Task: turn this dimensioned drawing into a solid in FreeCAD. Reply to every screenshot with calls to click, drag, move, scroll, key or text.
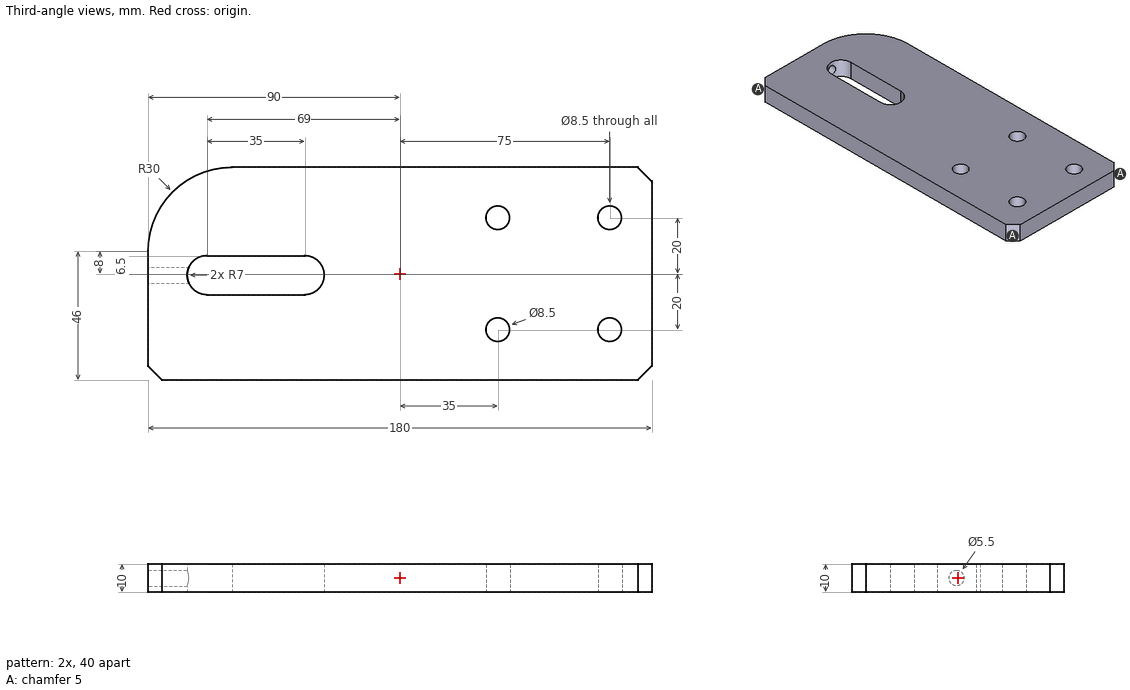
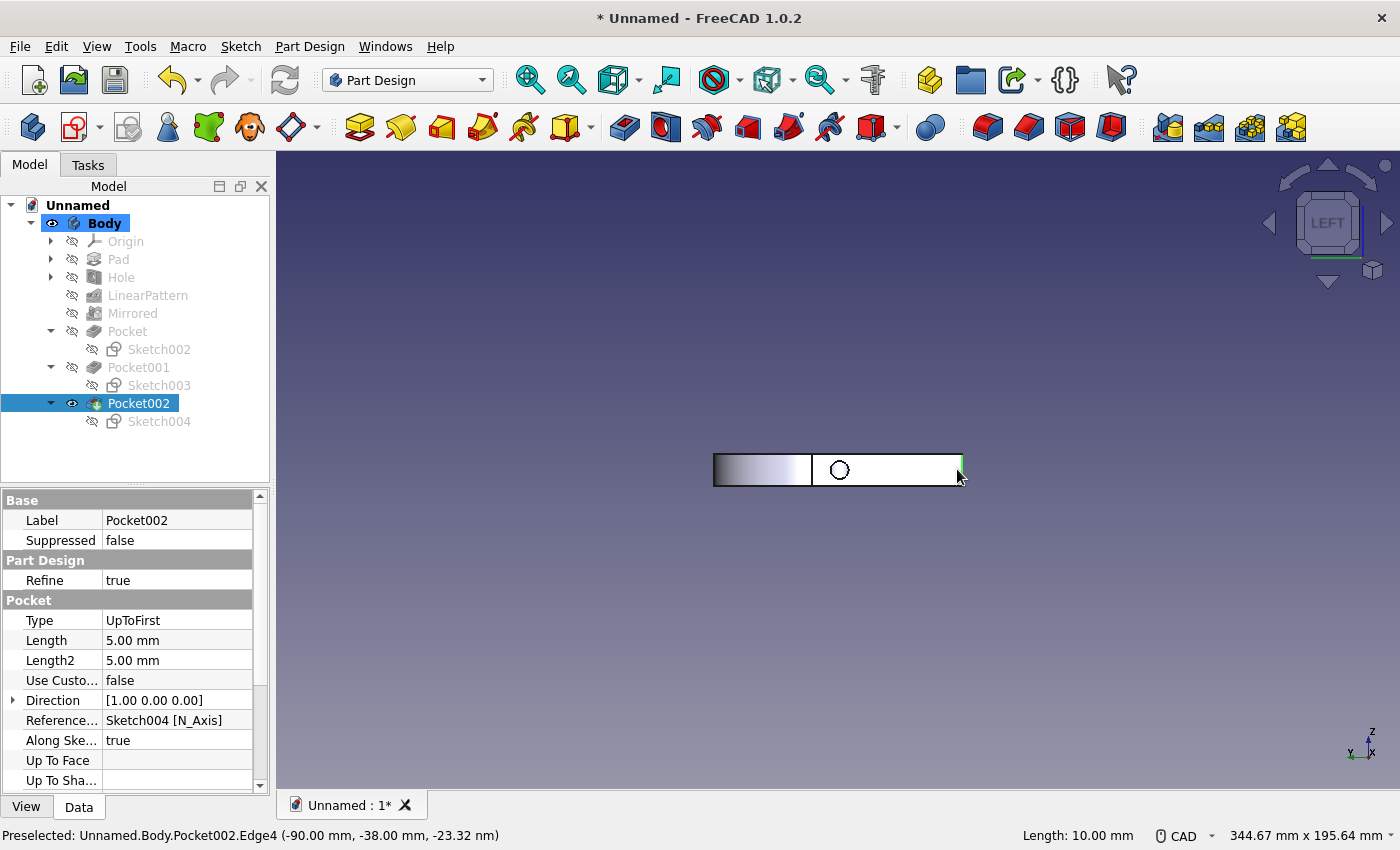
key(0)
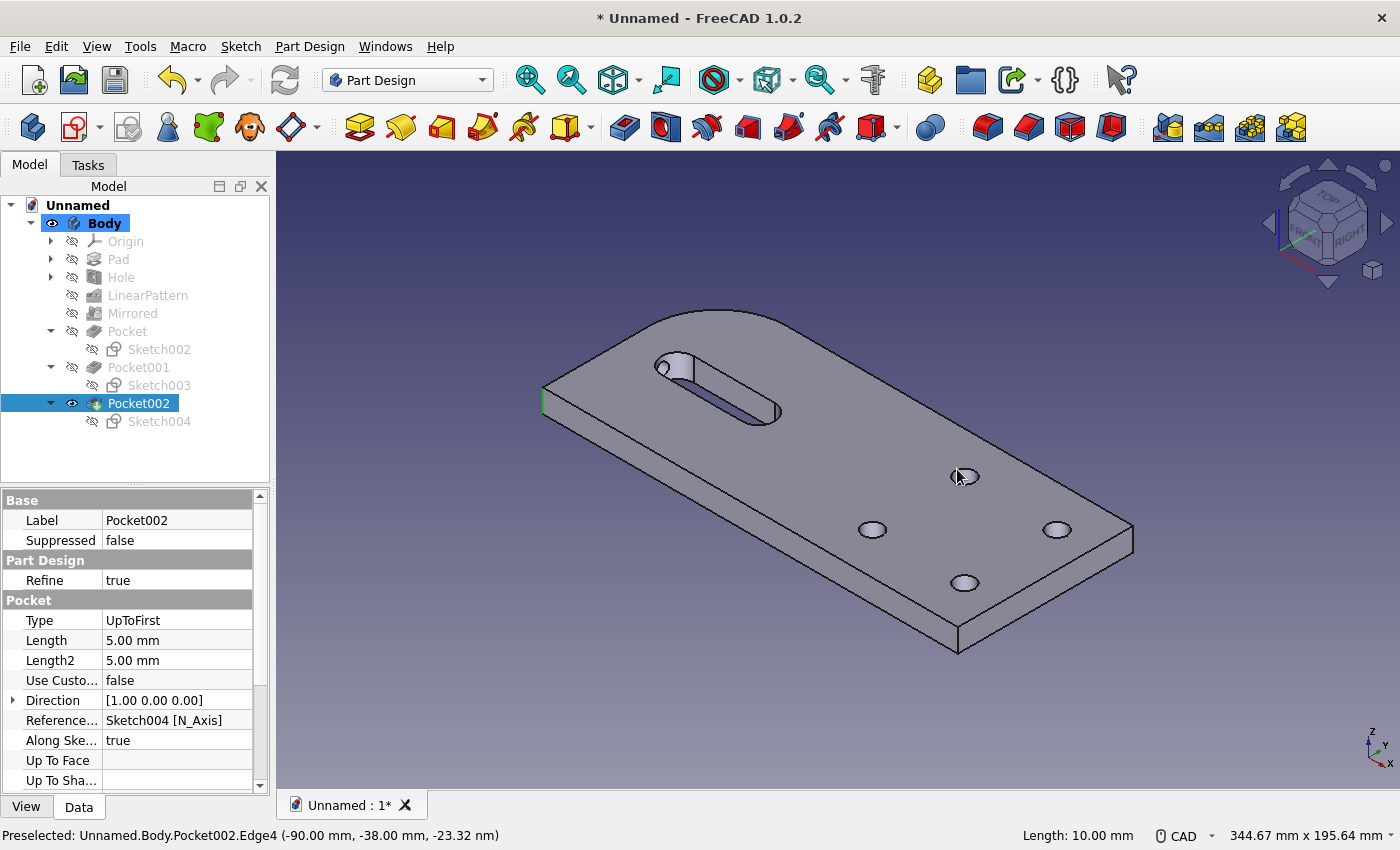
click(958, 639, ctrl)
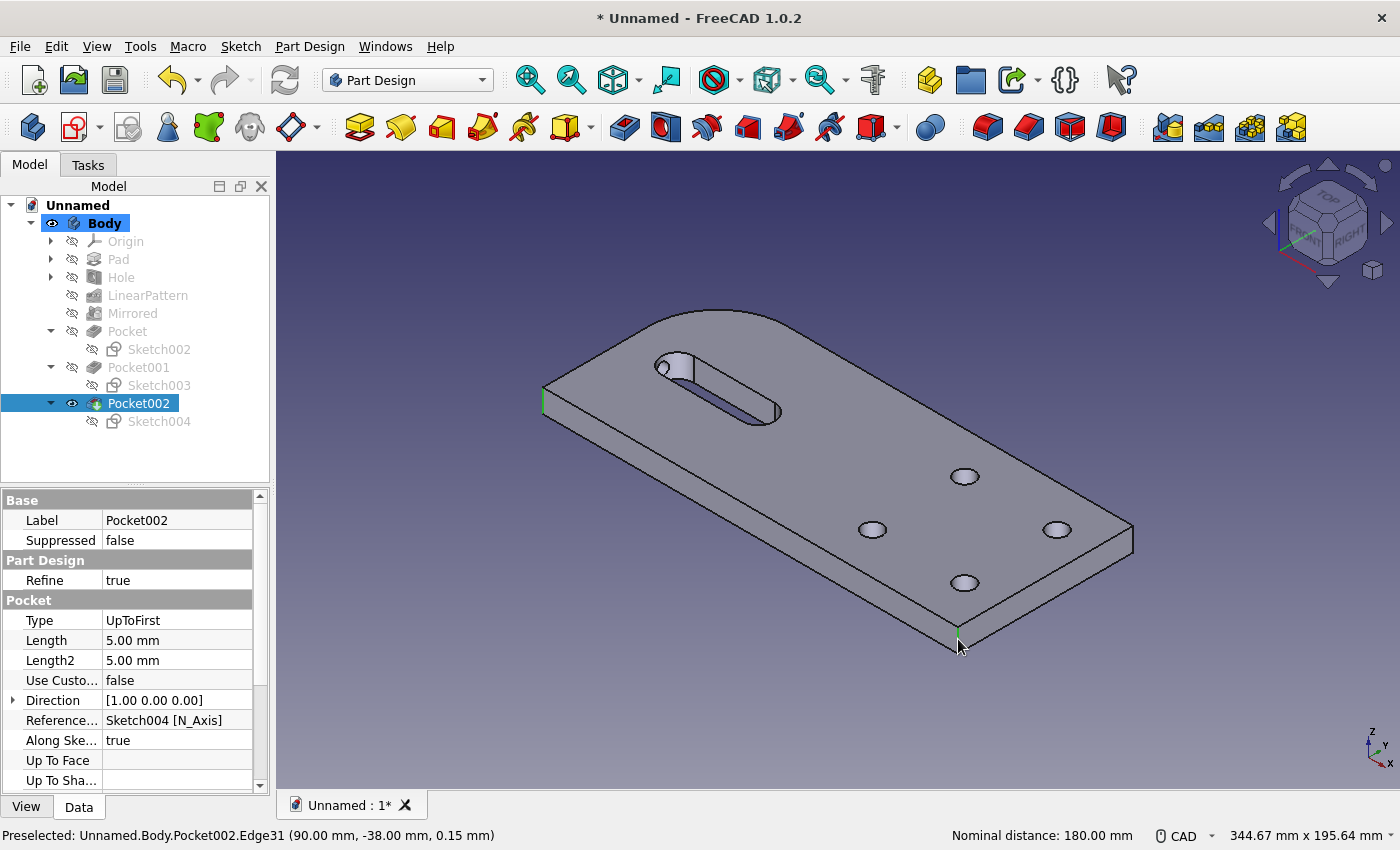
key(2)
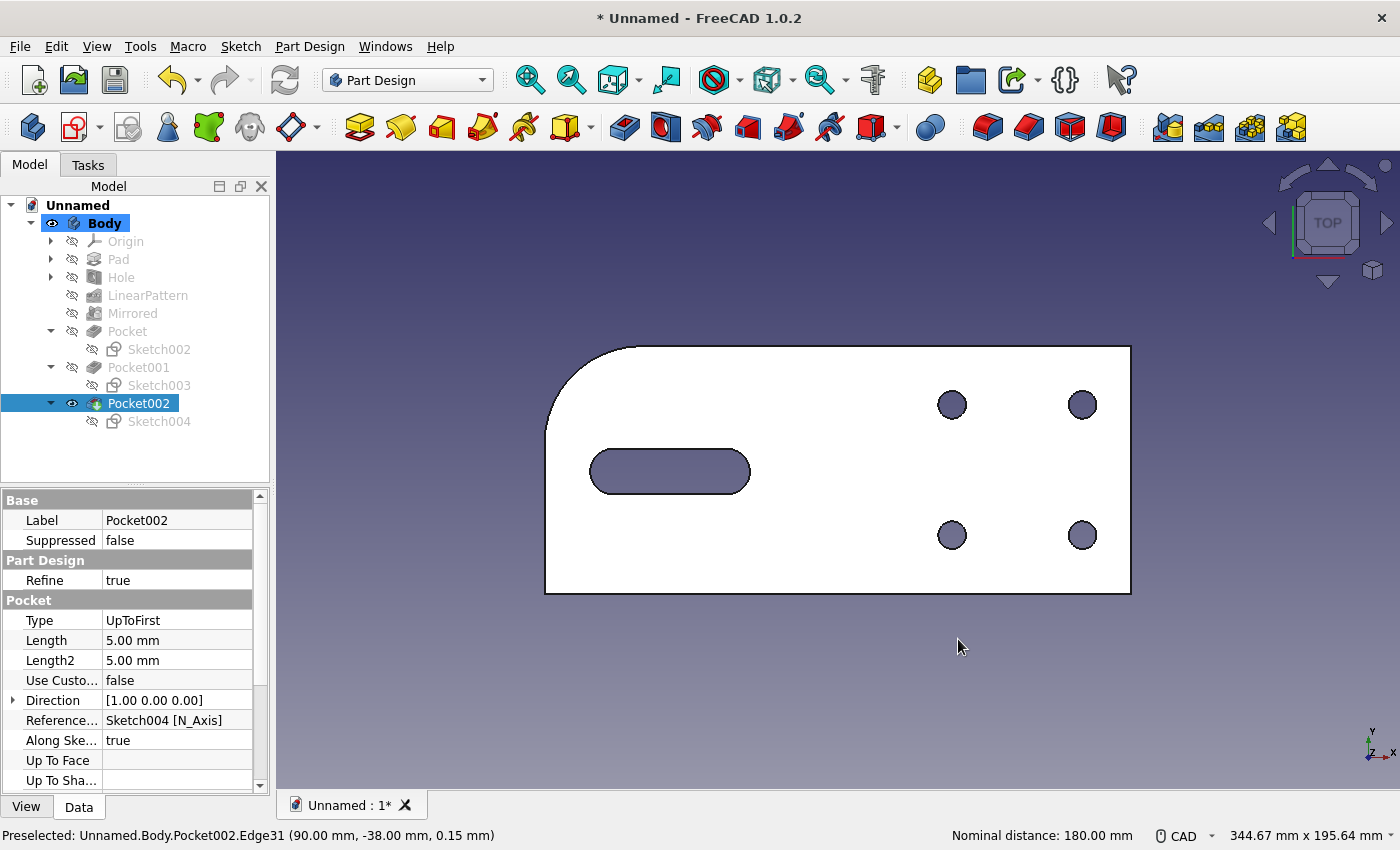
key(1)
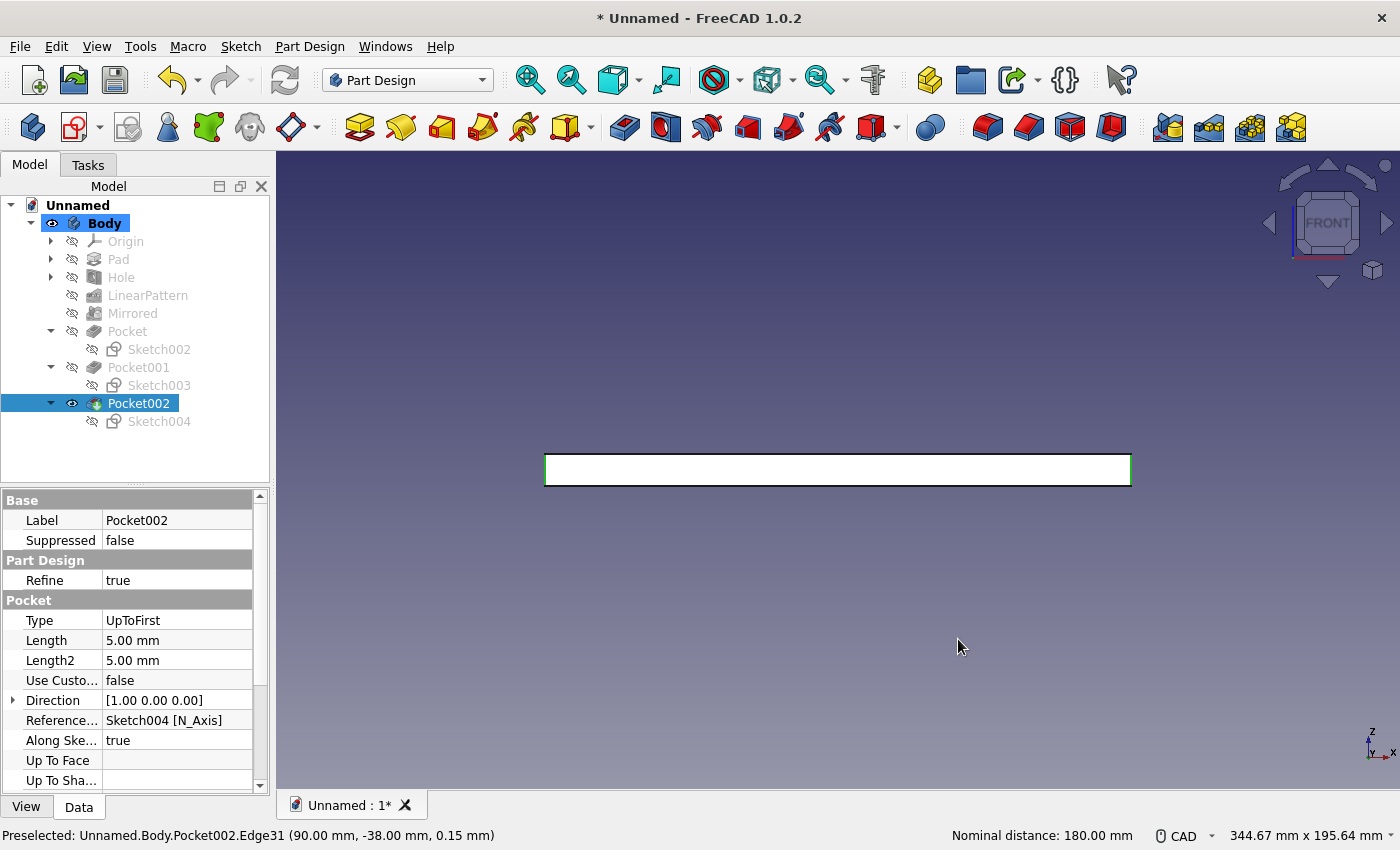
key(3)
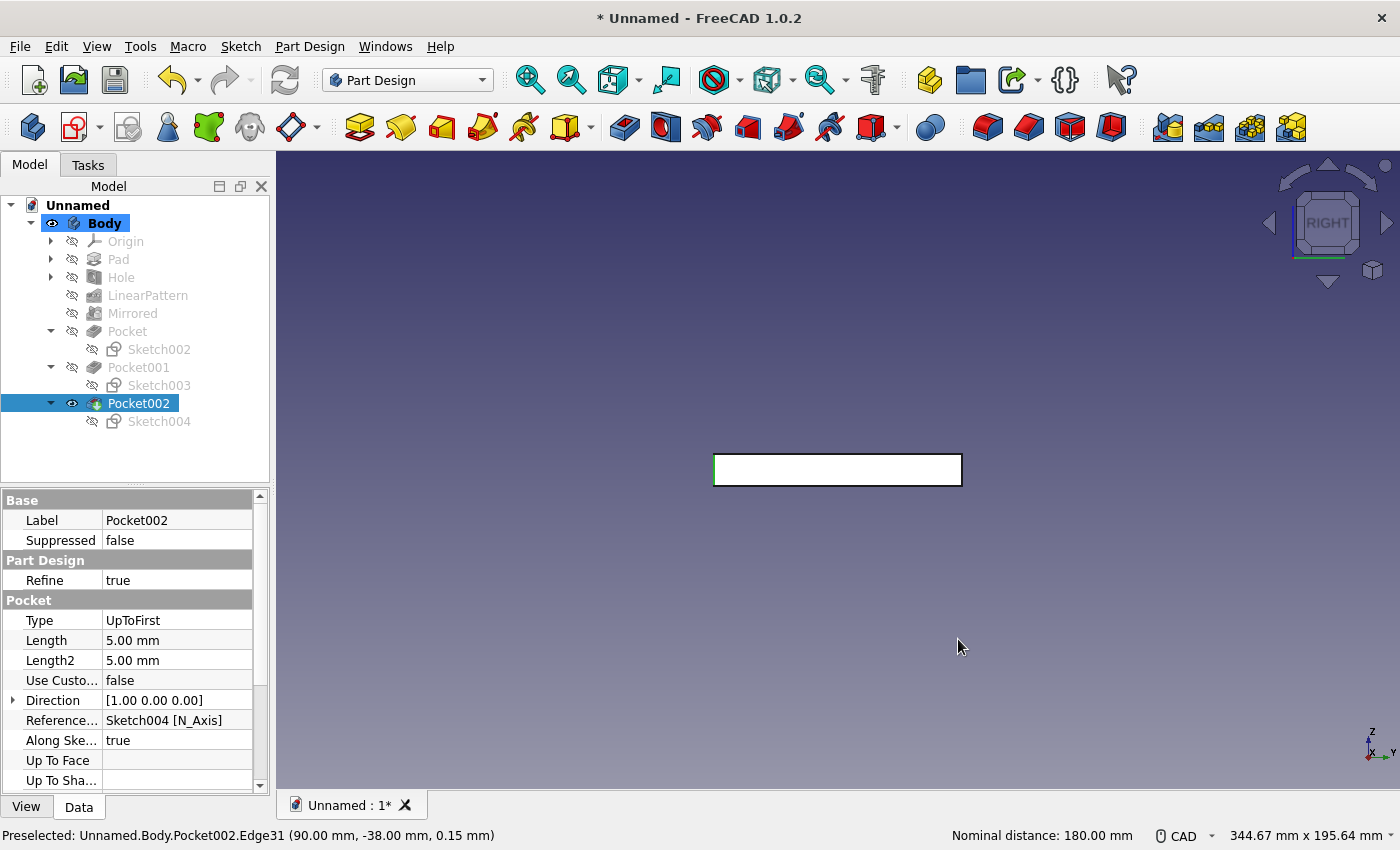
click(531, 80)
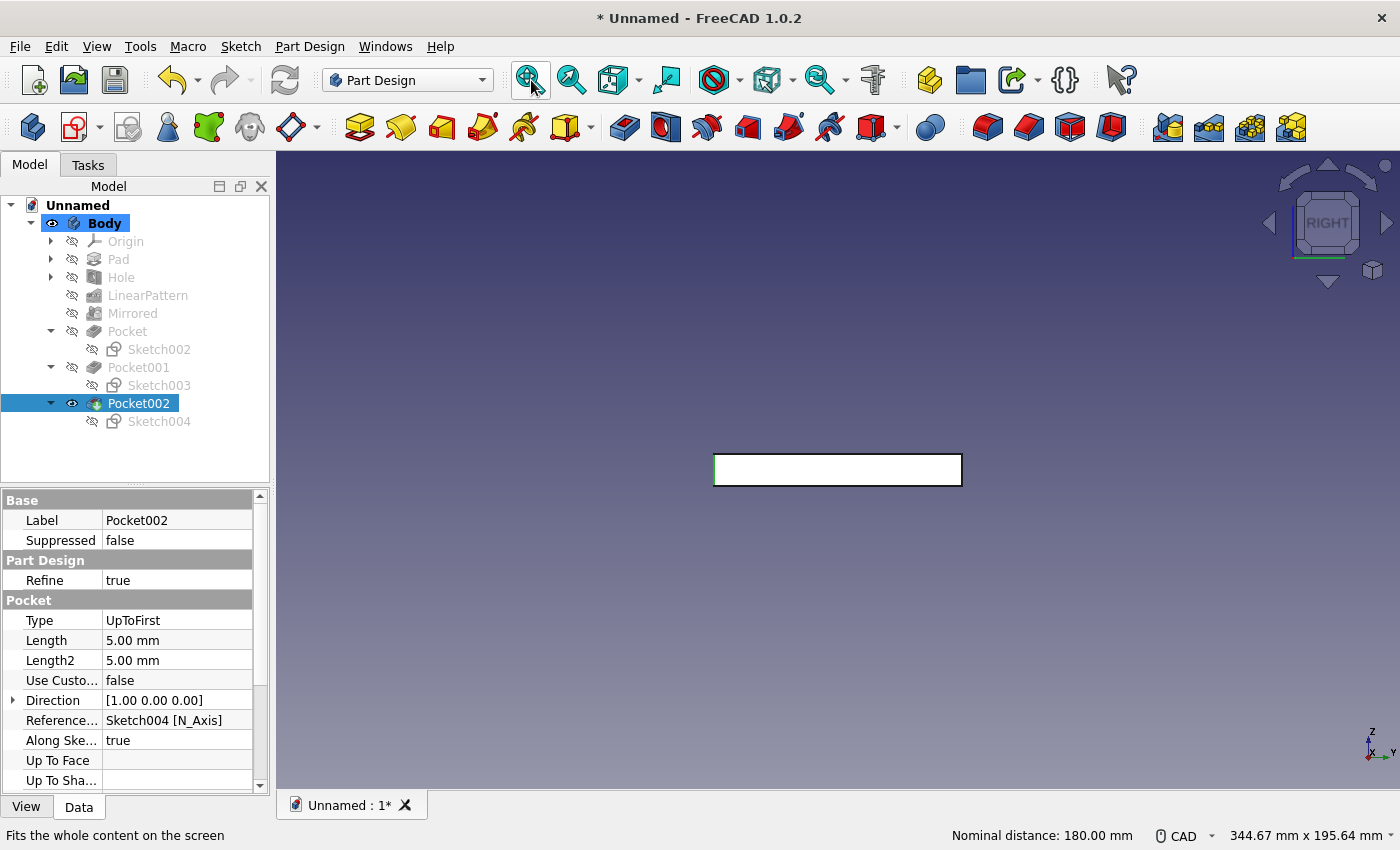
click(962, 469, ctrl)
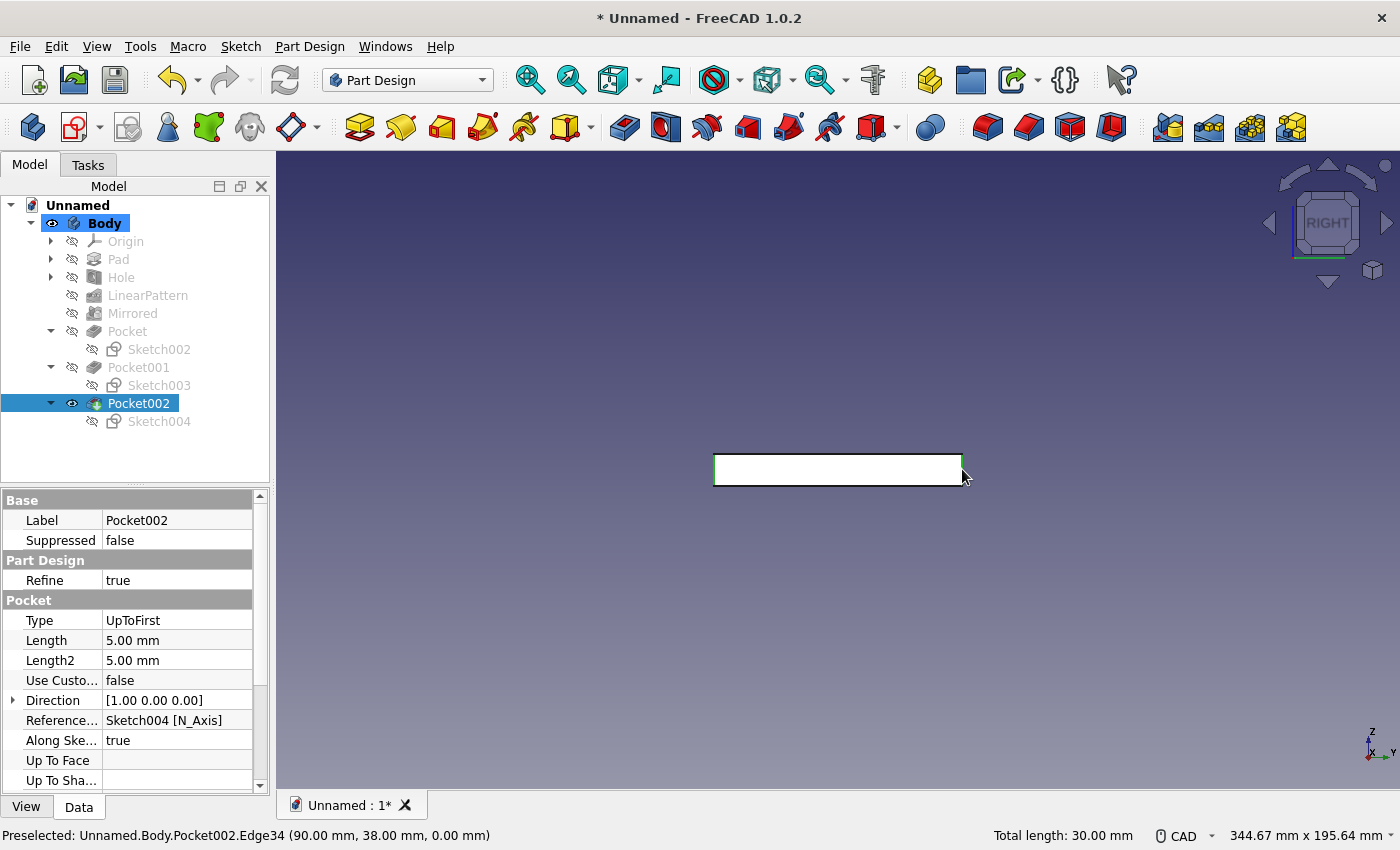
click(1029, 128)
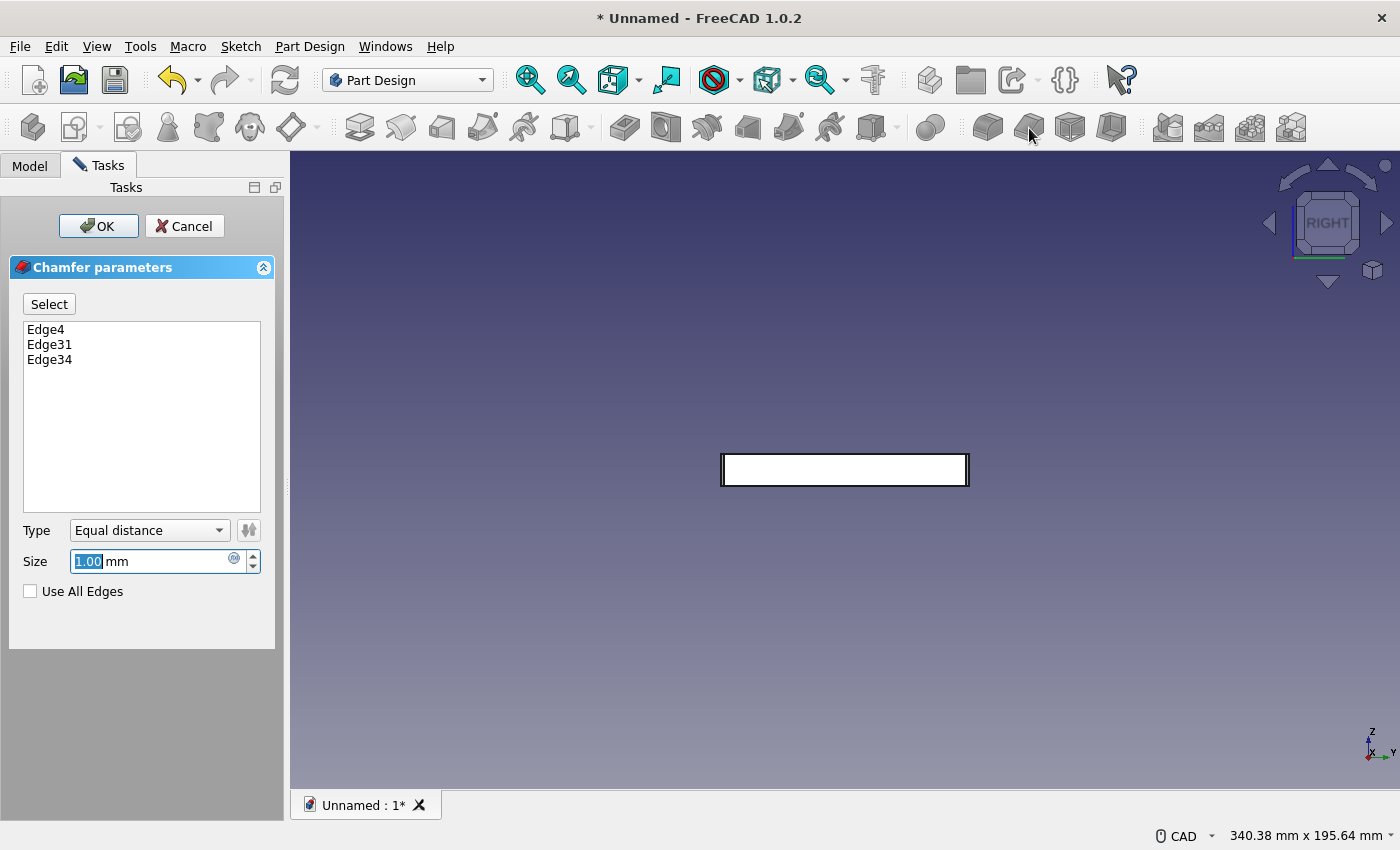
text(5)
key(Tab)